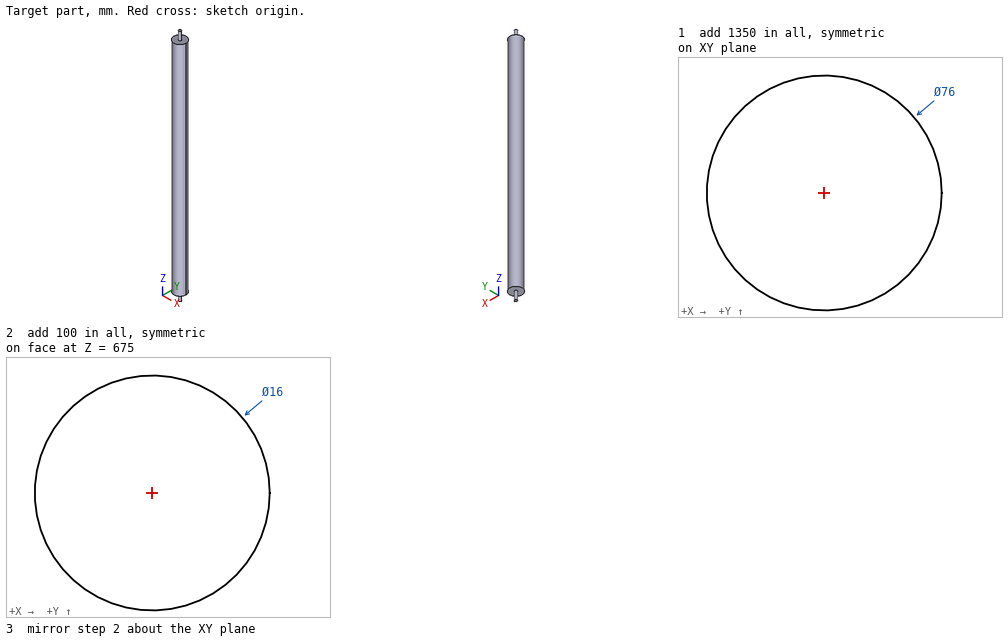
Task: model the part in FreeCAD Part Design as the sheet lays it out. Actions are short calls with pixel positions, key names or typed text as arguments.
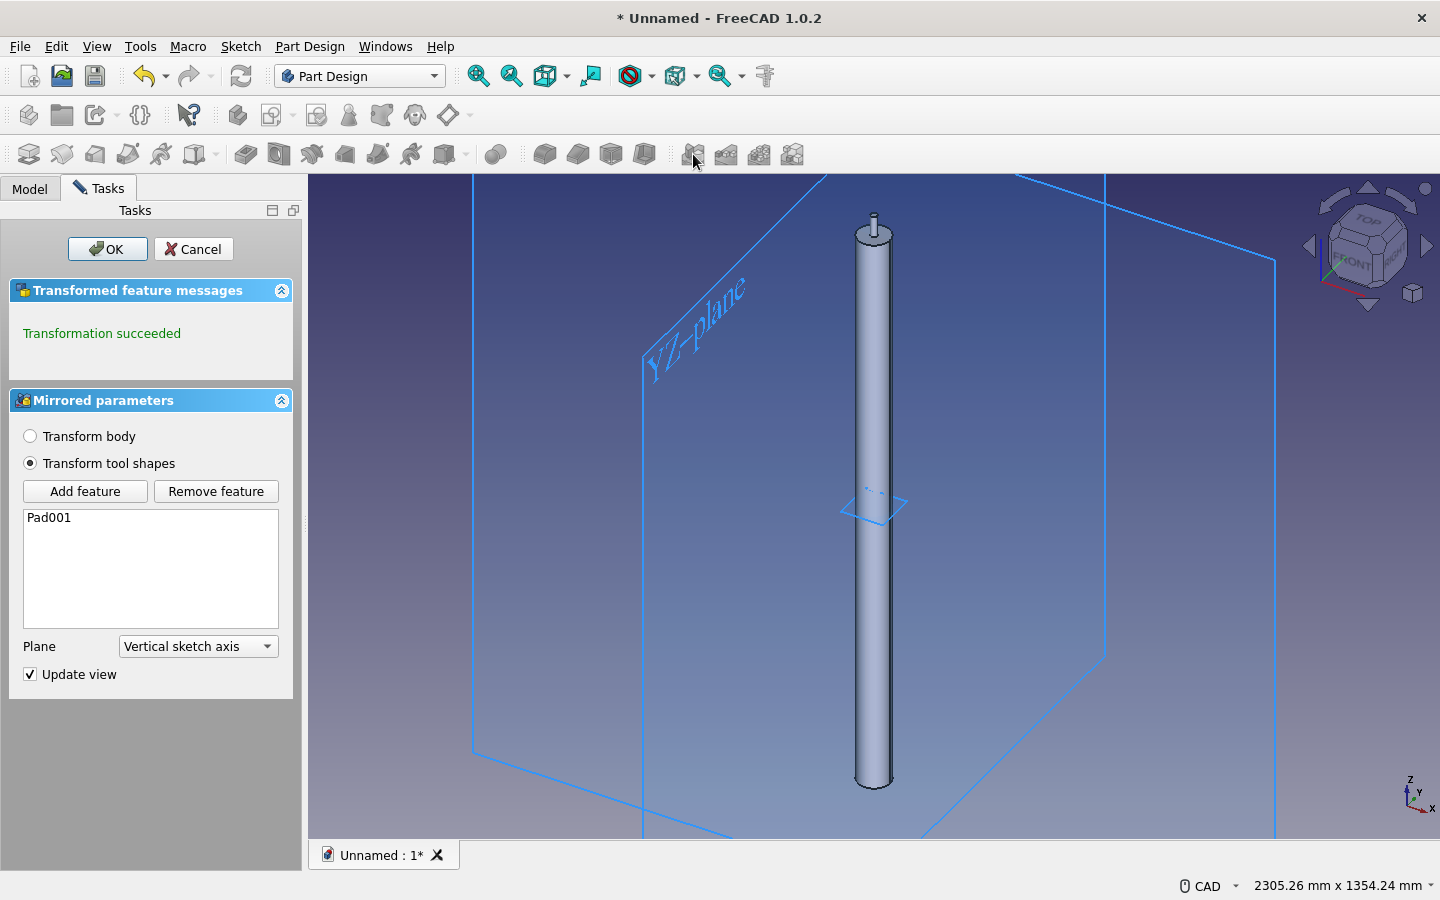
click(199, 646)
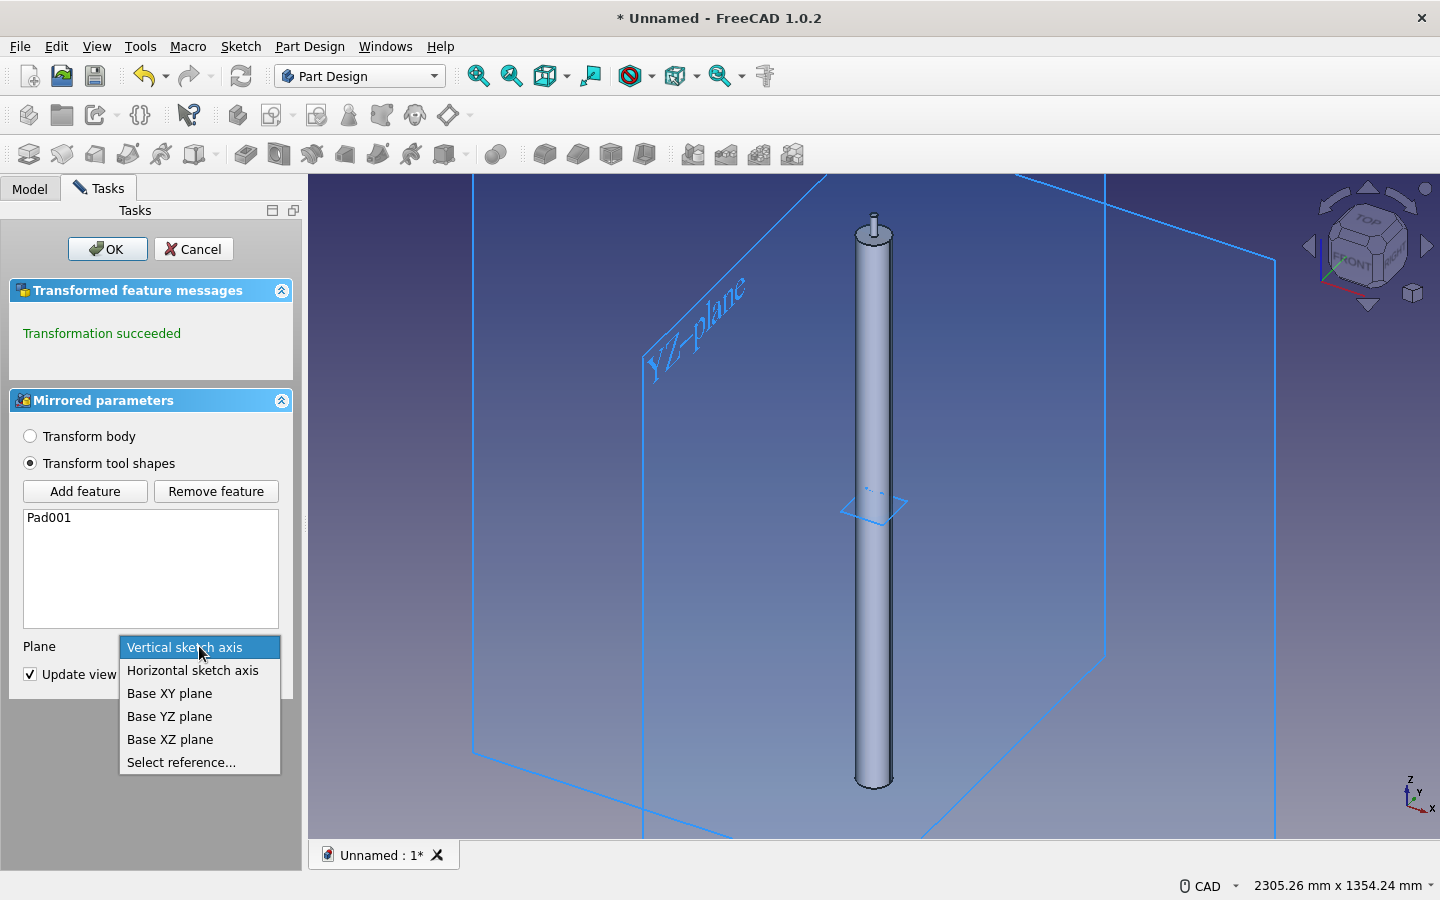
click(198, 694)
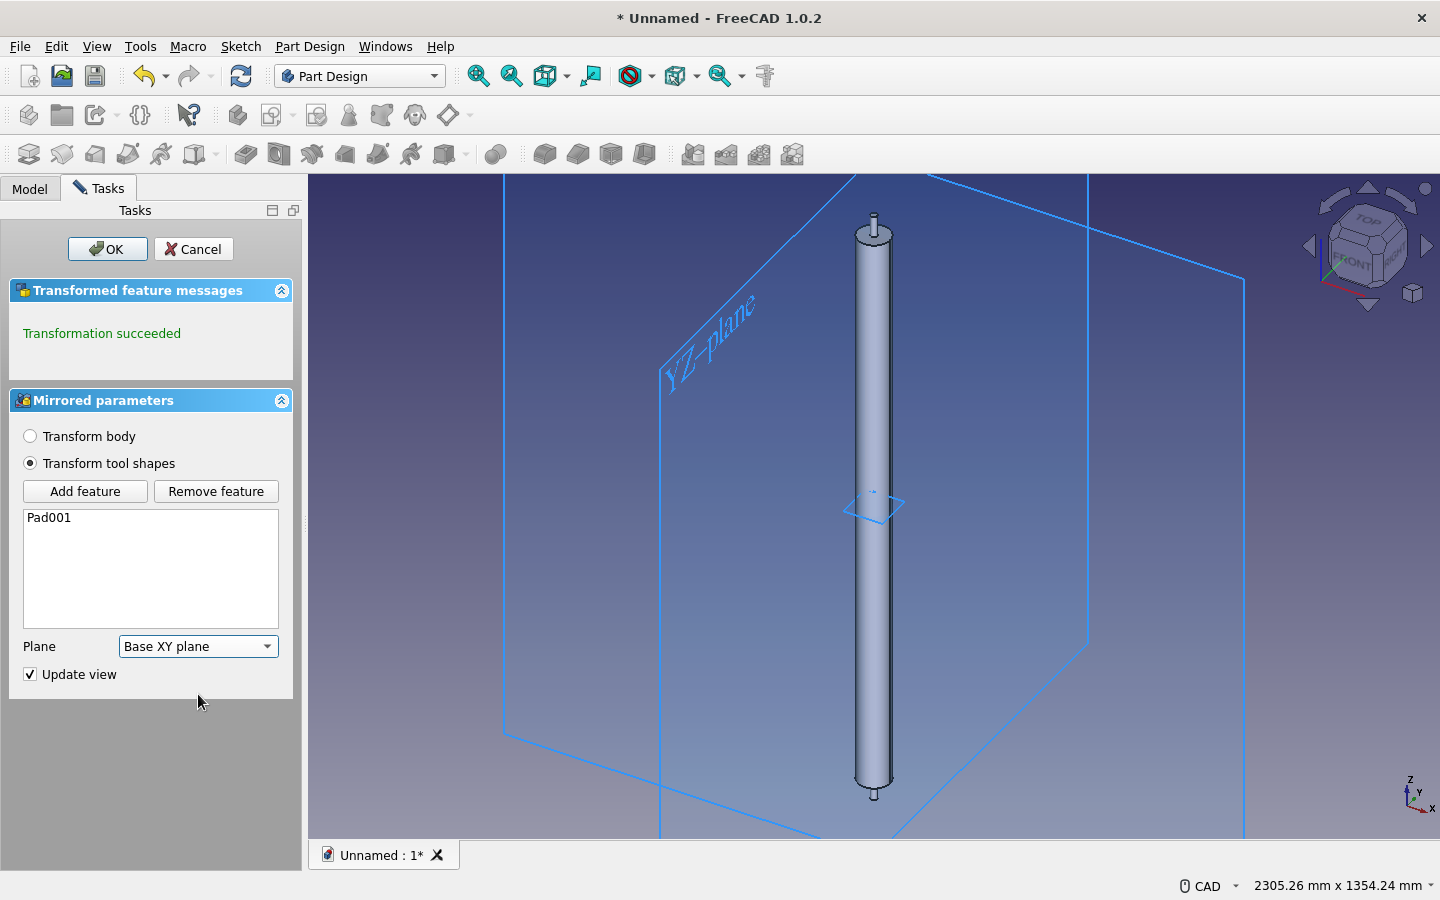
click(108, 249)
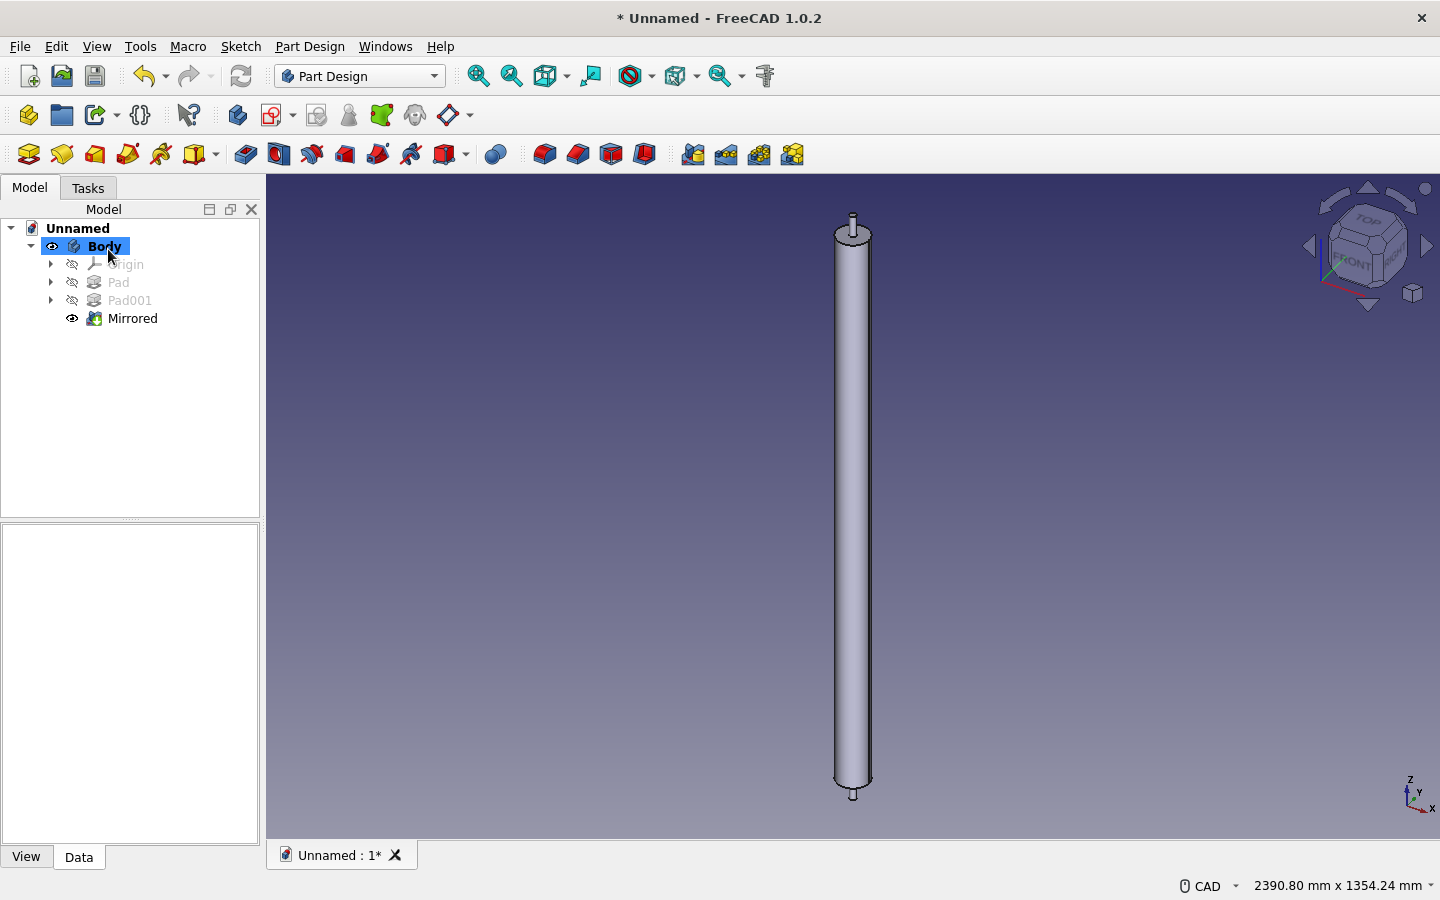
key(0)